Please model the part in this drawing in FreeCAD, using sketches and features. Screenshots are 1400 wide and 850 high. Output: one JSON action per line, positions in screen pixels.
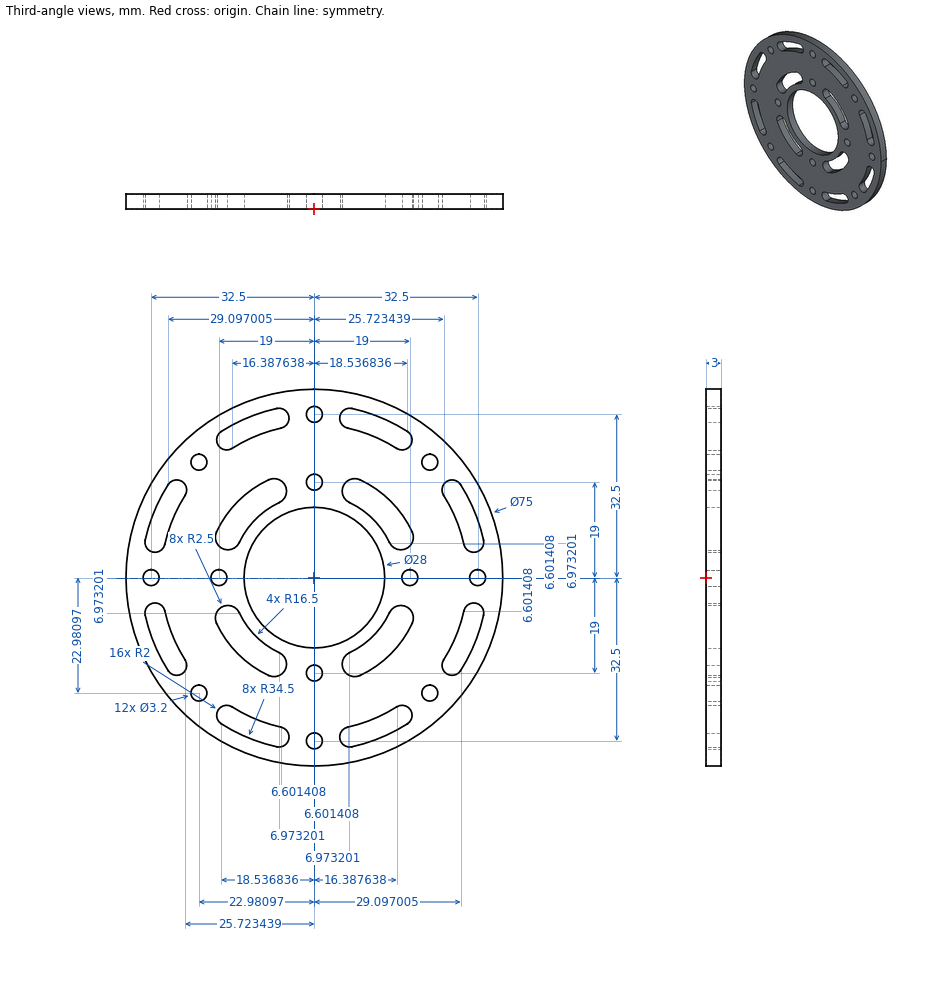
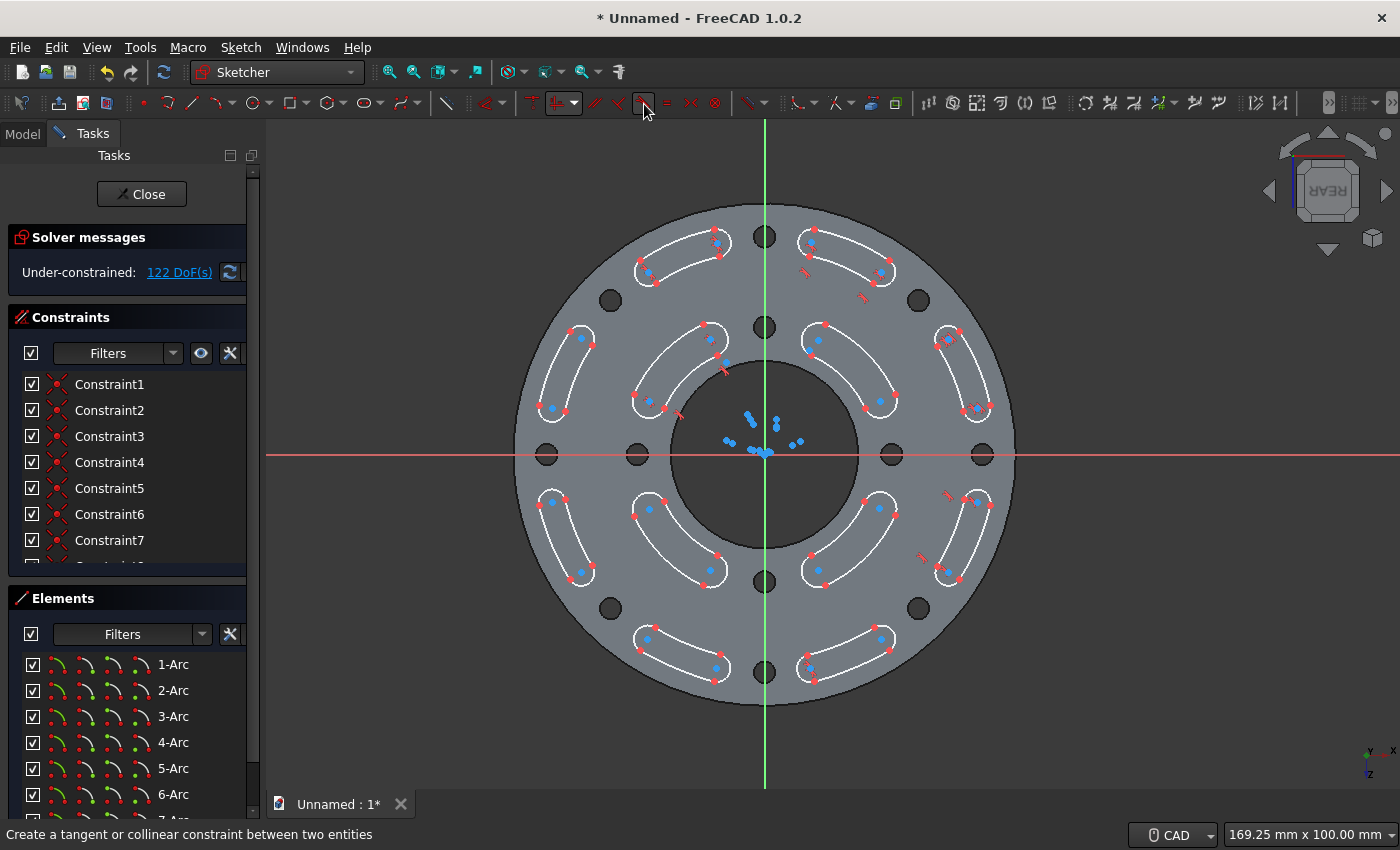
{"action": "left_click", "coordinate": [838, 674]}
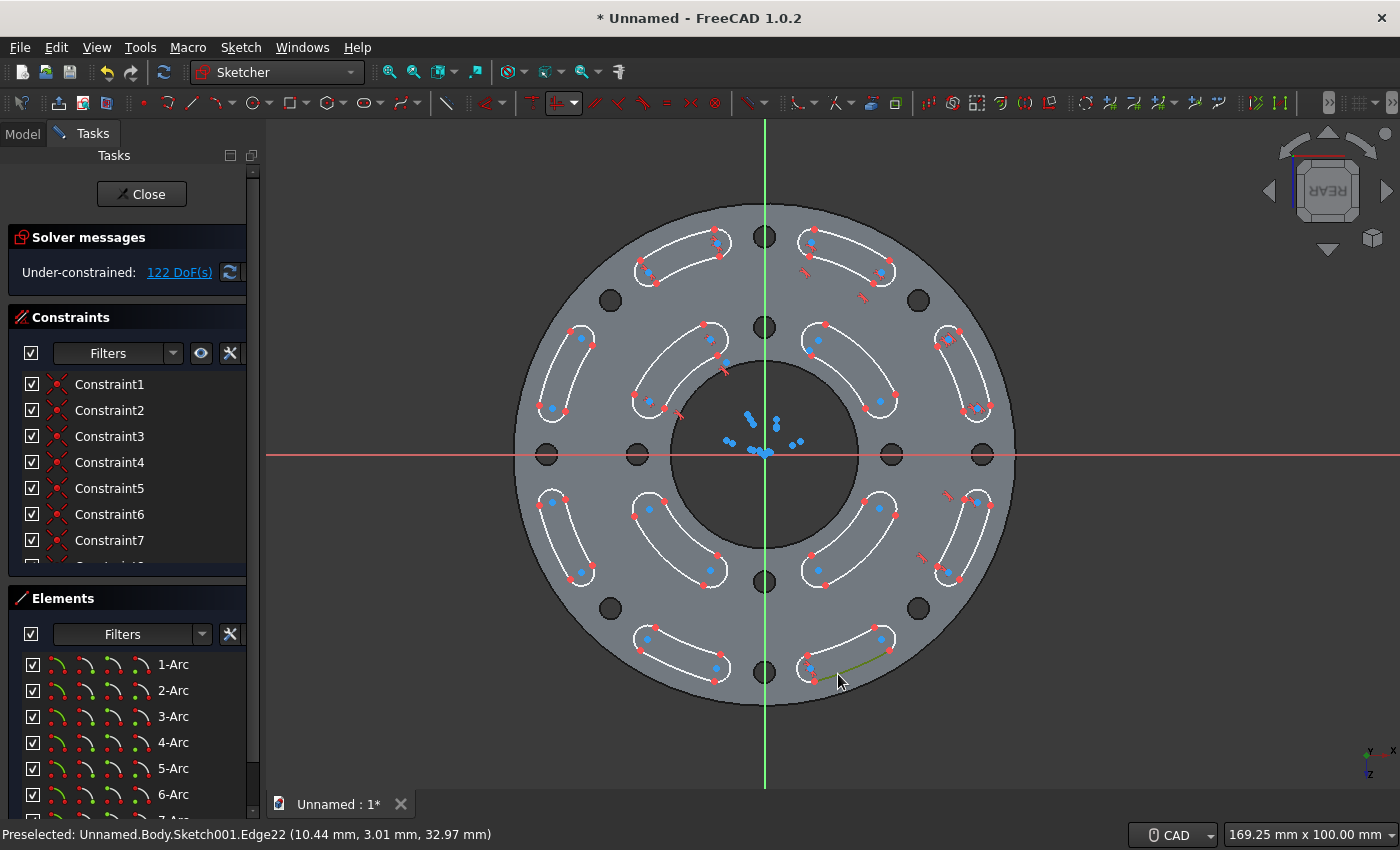
{"action": "left_click", "coordinate": [895, 640]}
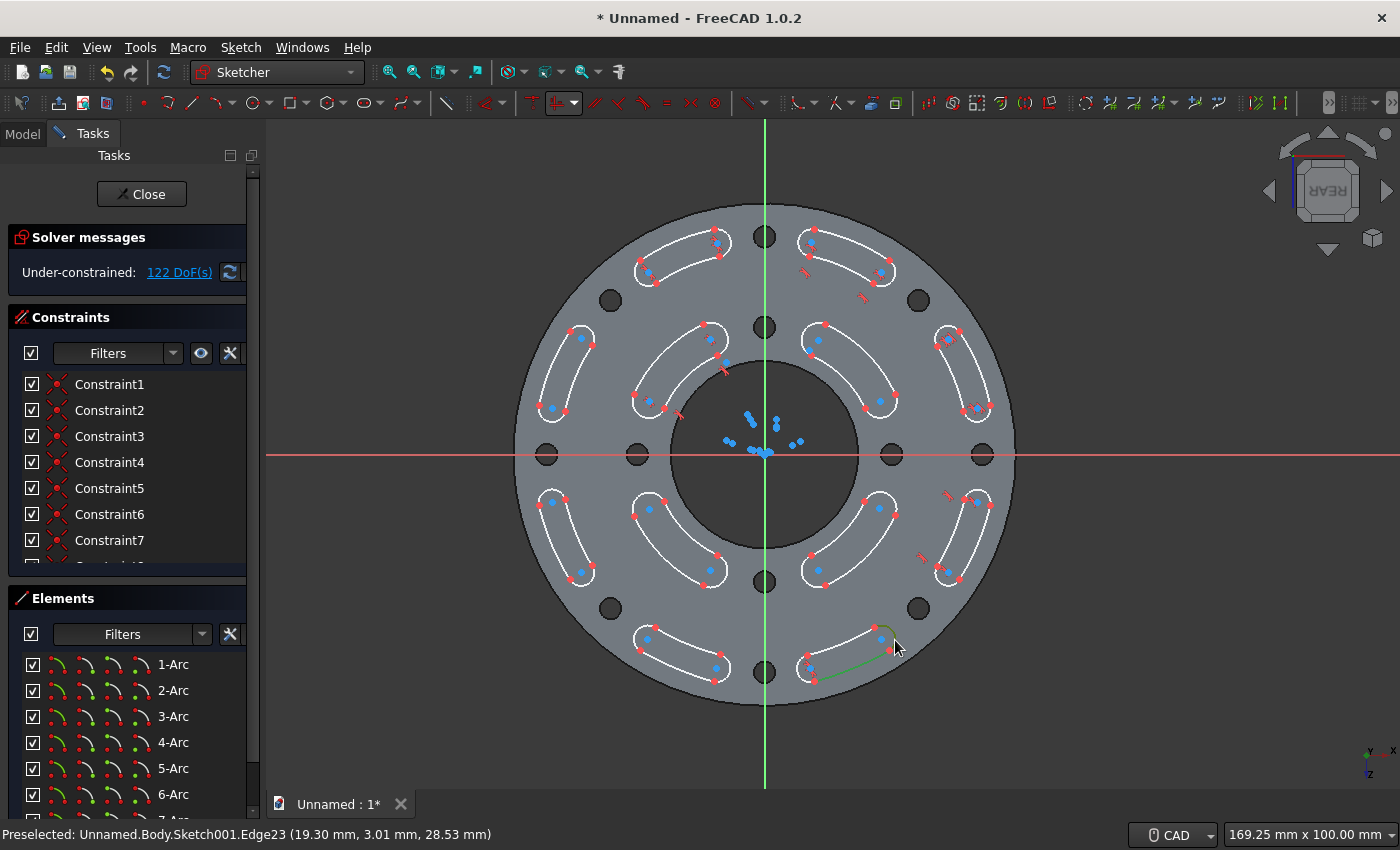
{"action": "left_click", "coordinate": [644, 104]}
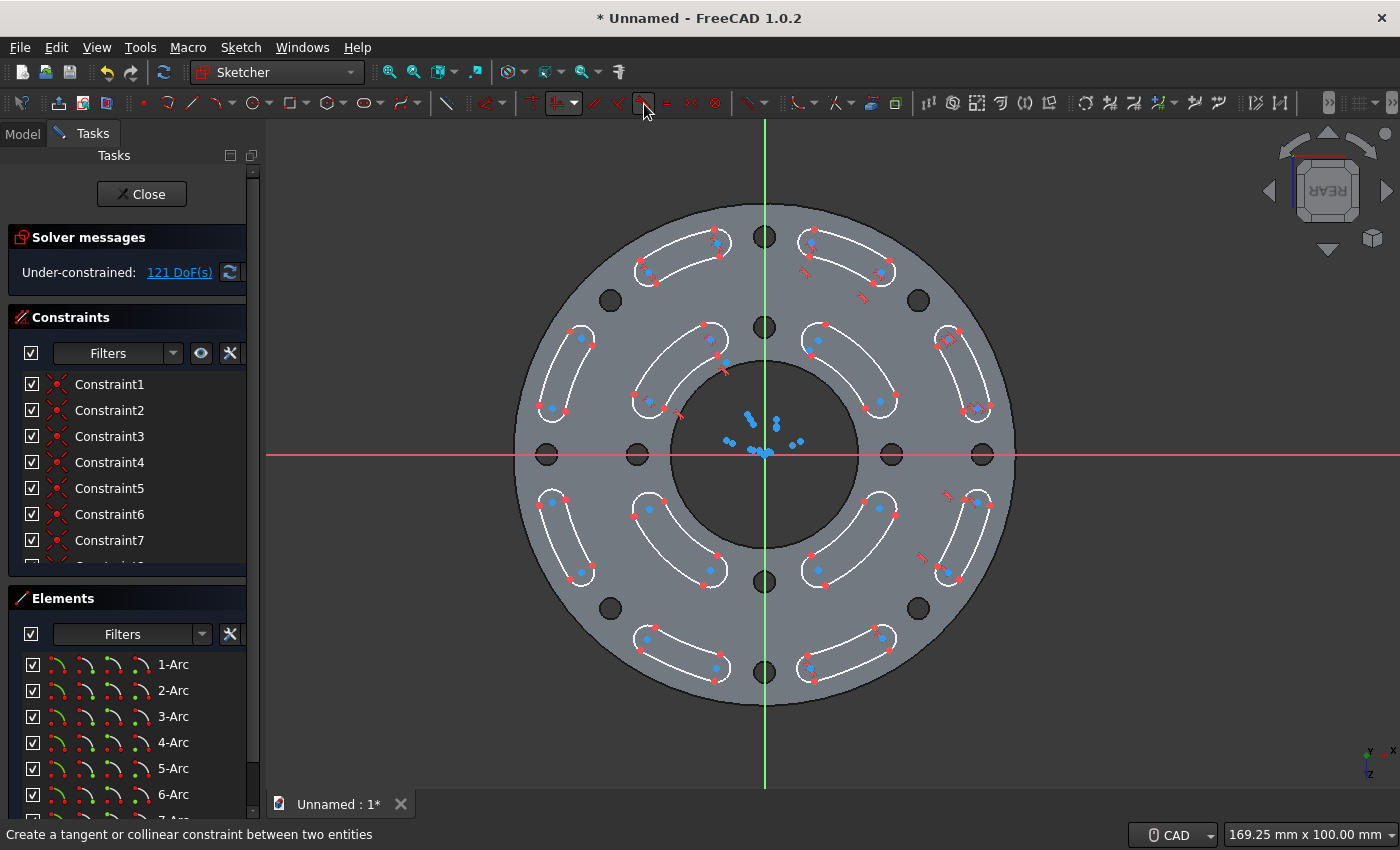
{"action": "left_click", "coordinate": [896, 640]}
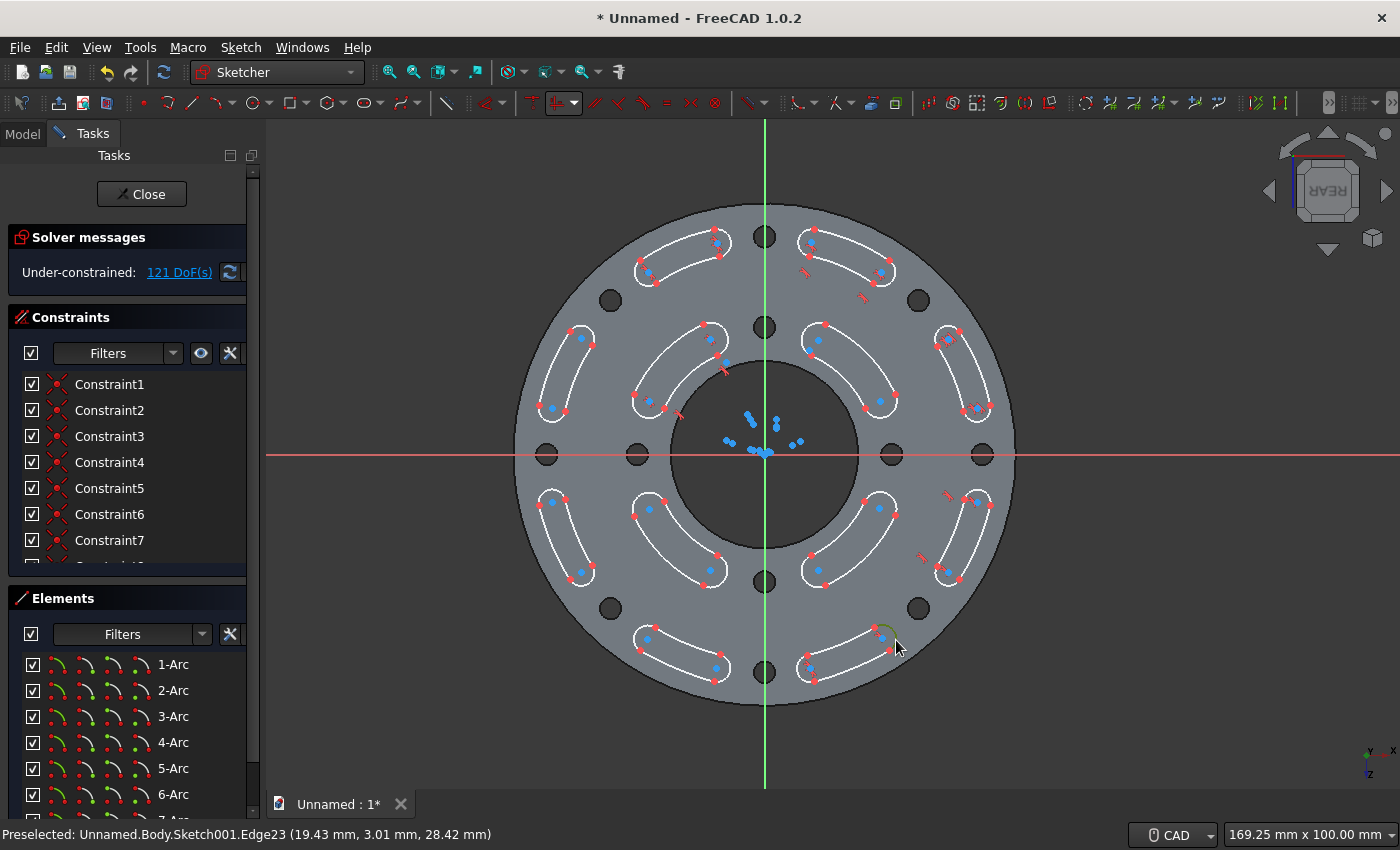
{"action": "left_click", "coordinate": [828, 649]}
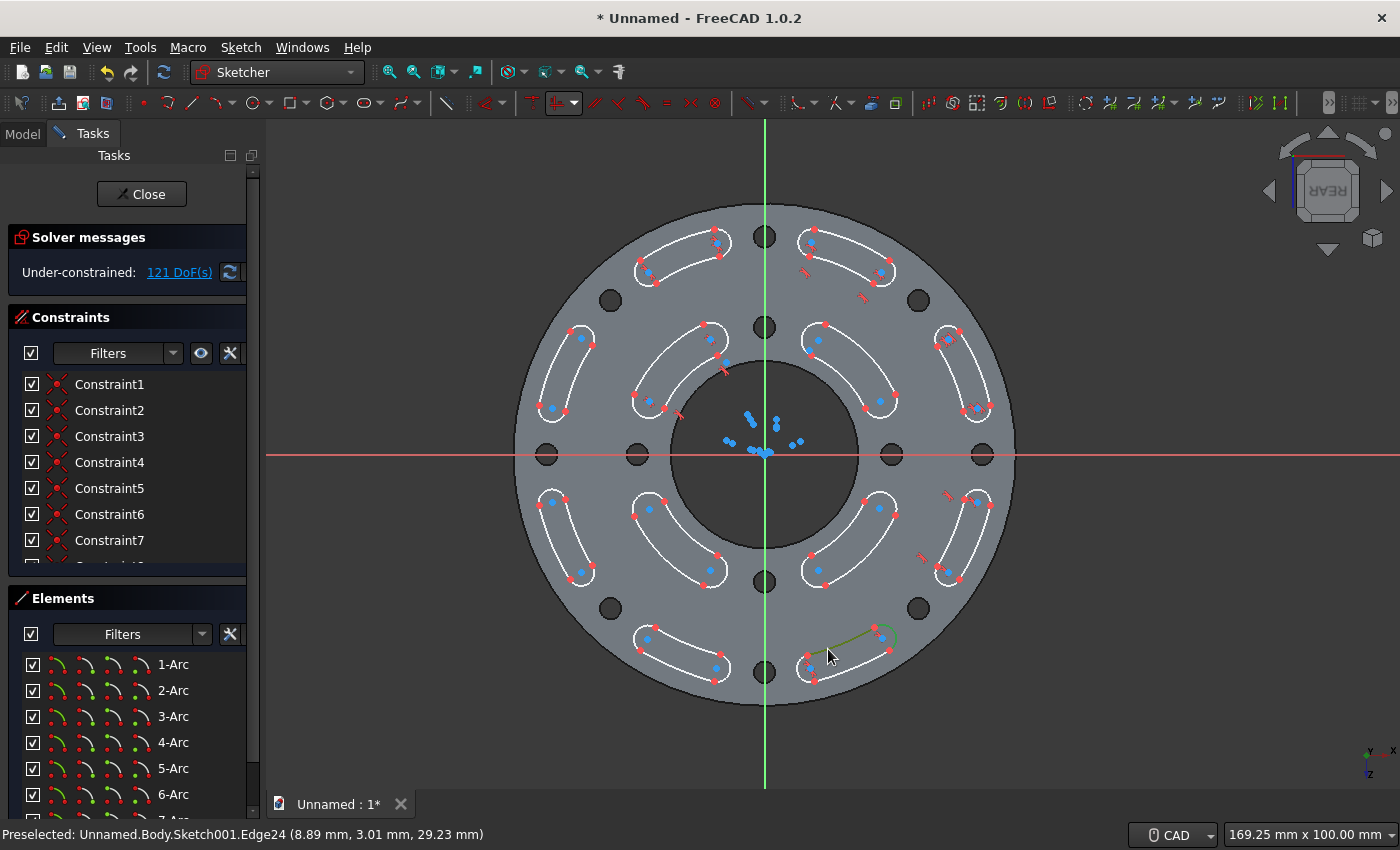
{"action": "left_click", "coordinate": [644, 104]}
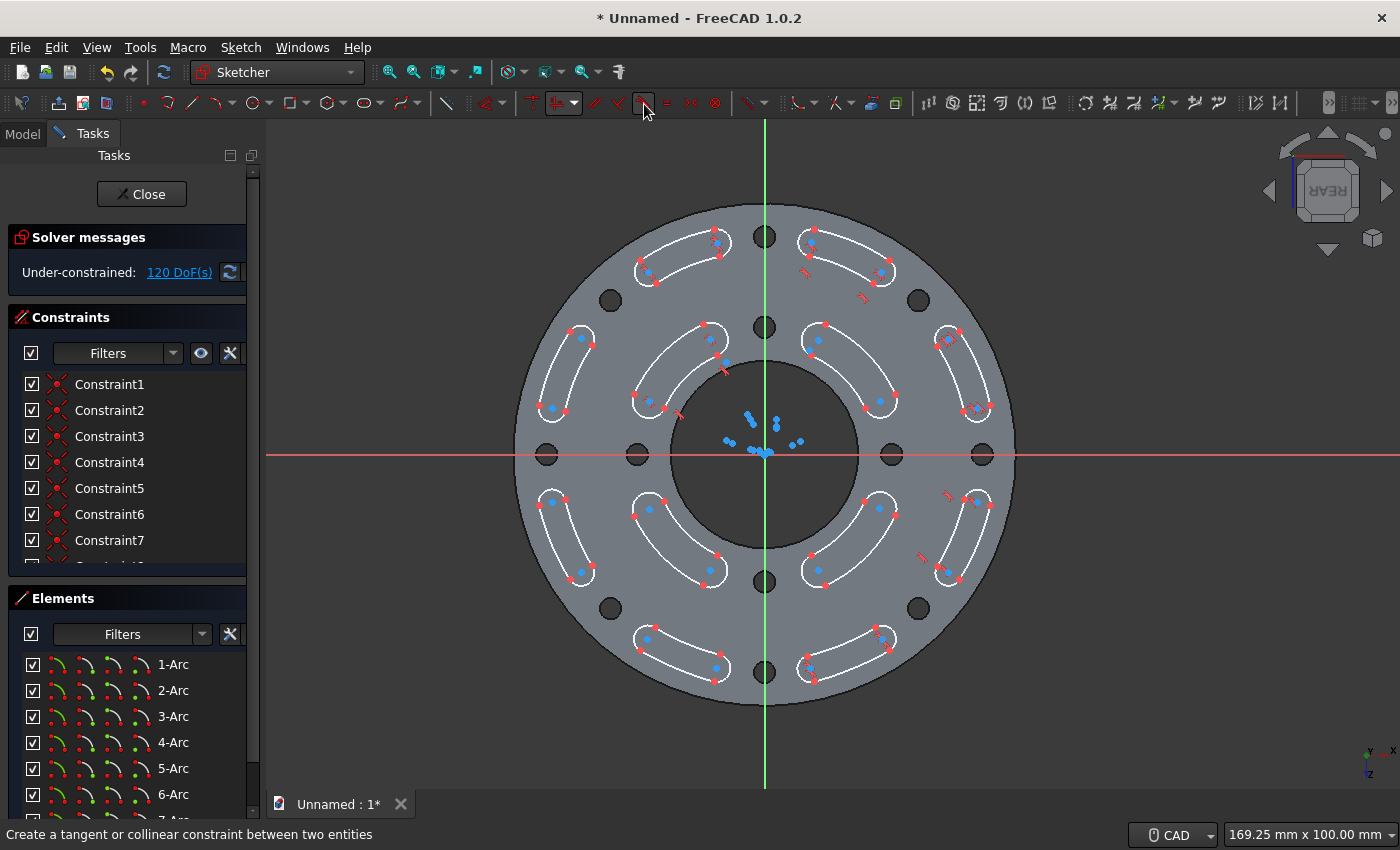
{"action": "left_click", "coordinate": [674, 638]}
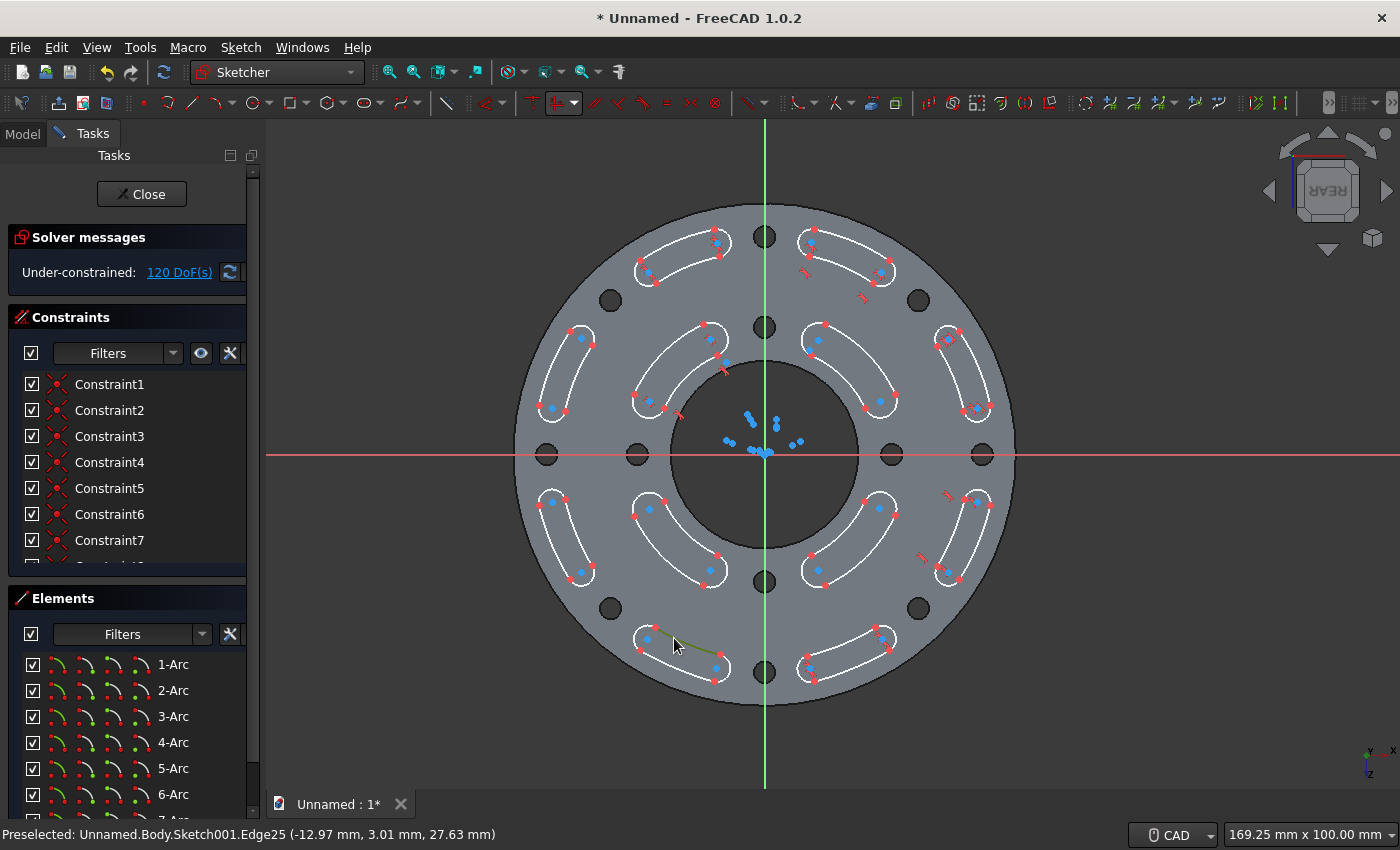
{"action": "left_click", "coordinate": [643, 626]}